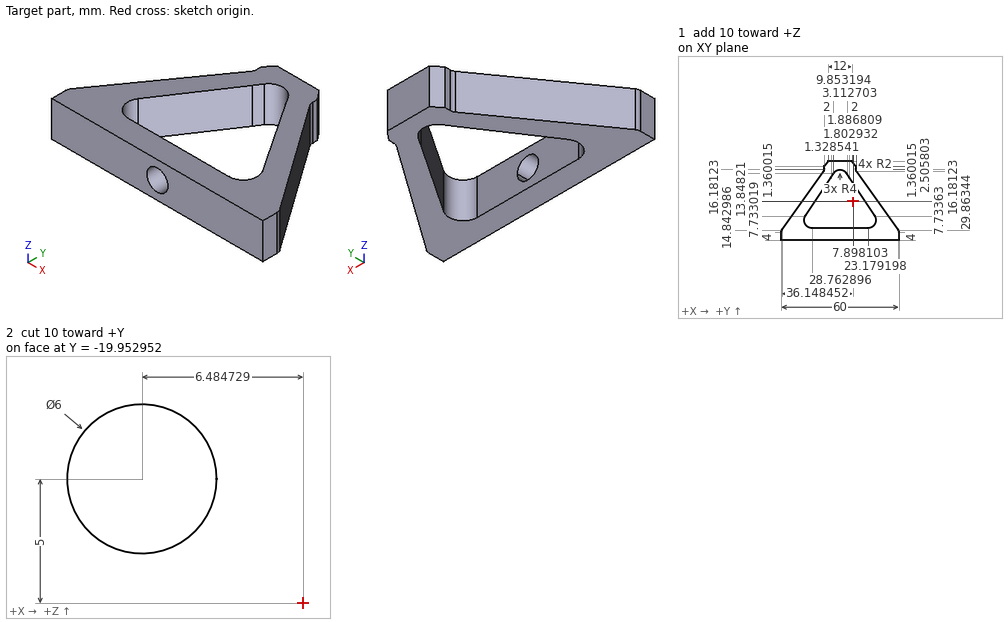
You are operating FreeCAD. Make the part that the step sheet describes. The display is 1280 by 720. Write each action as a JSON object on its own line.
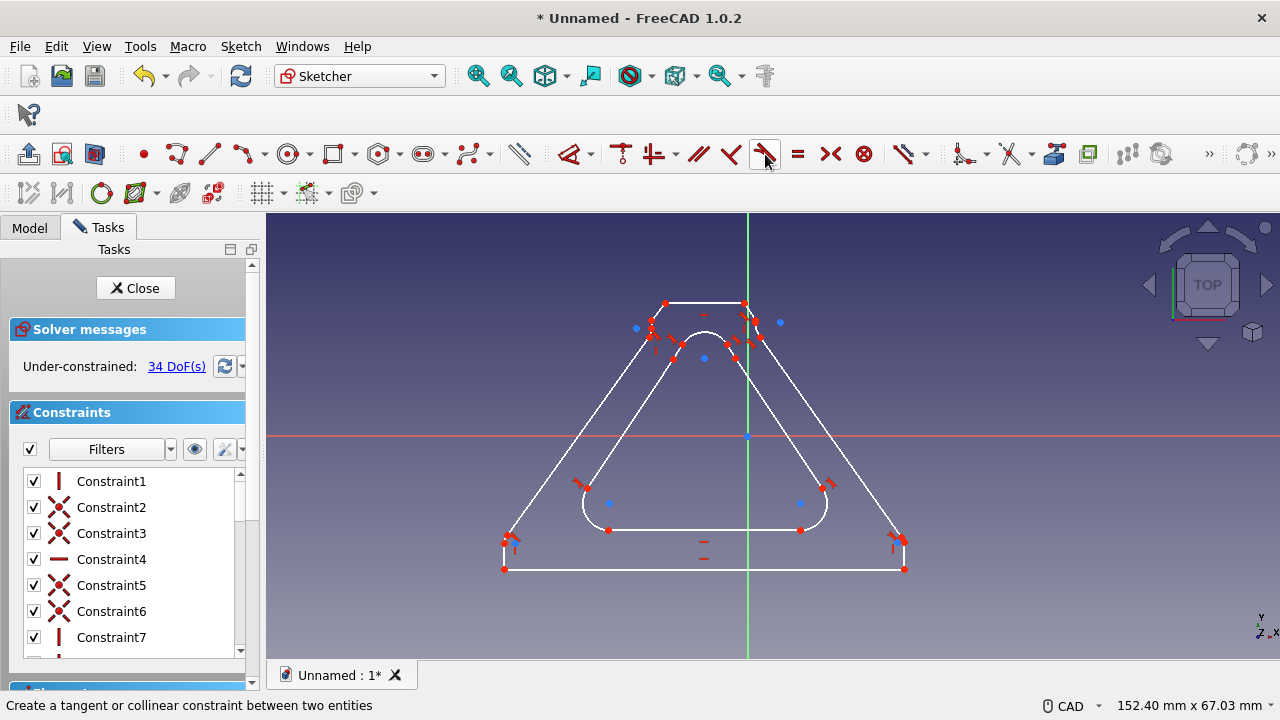
{"action": "left_click", "coordinate": [666, 530]}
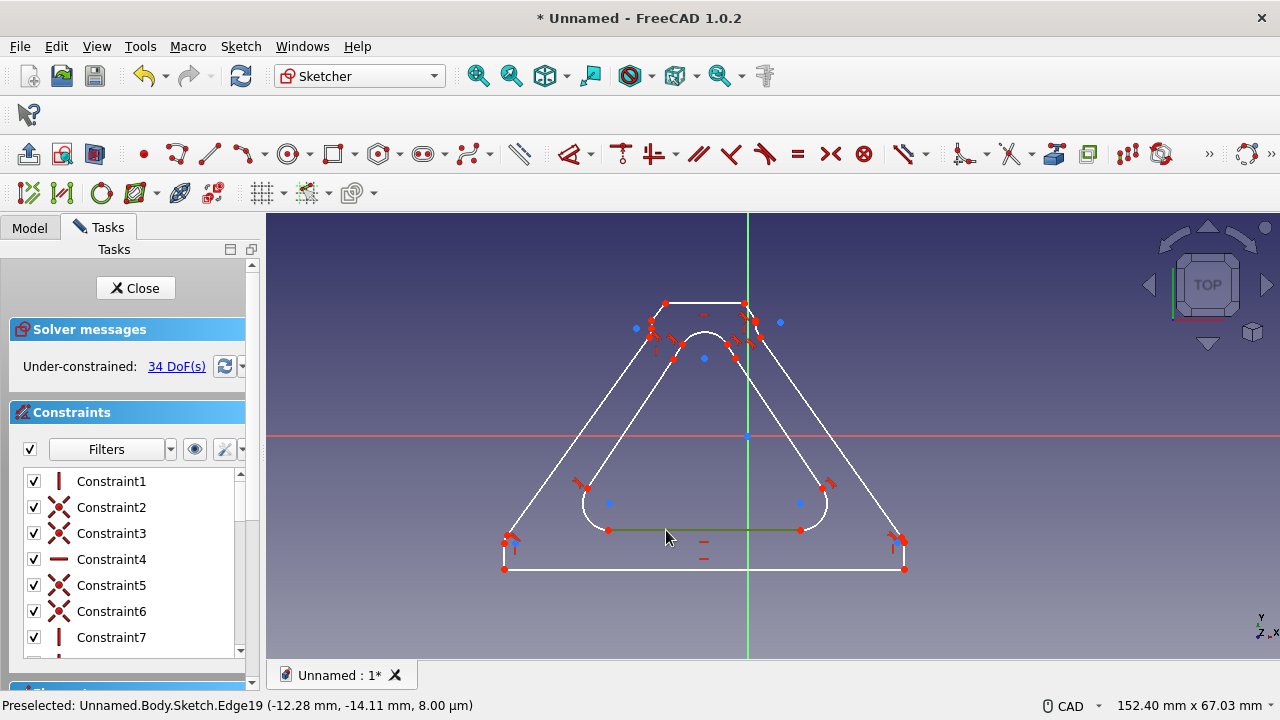
{"action": "left_click", "coordinate": [816, 525]}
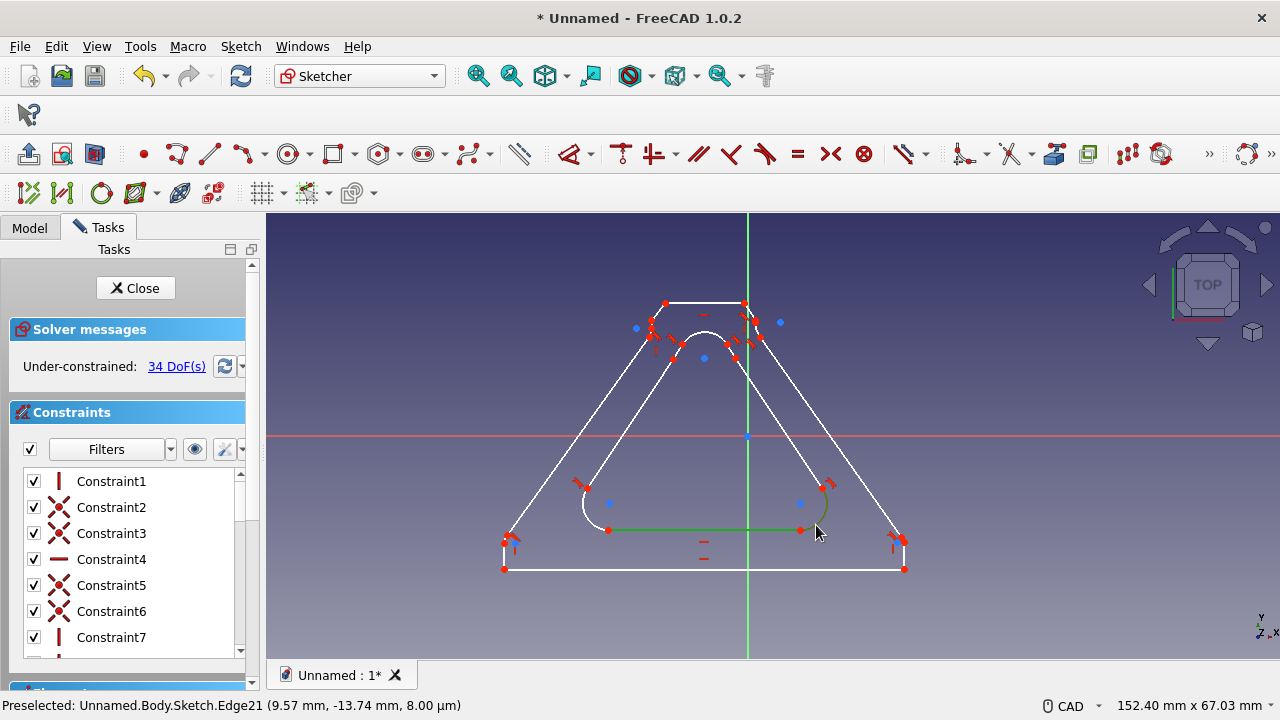
{"action": "left_click", "coordinate": [765, 154]}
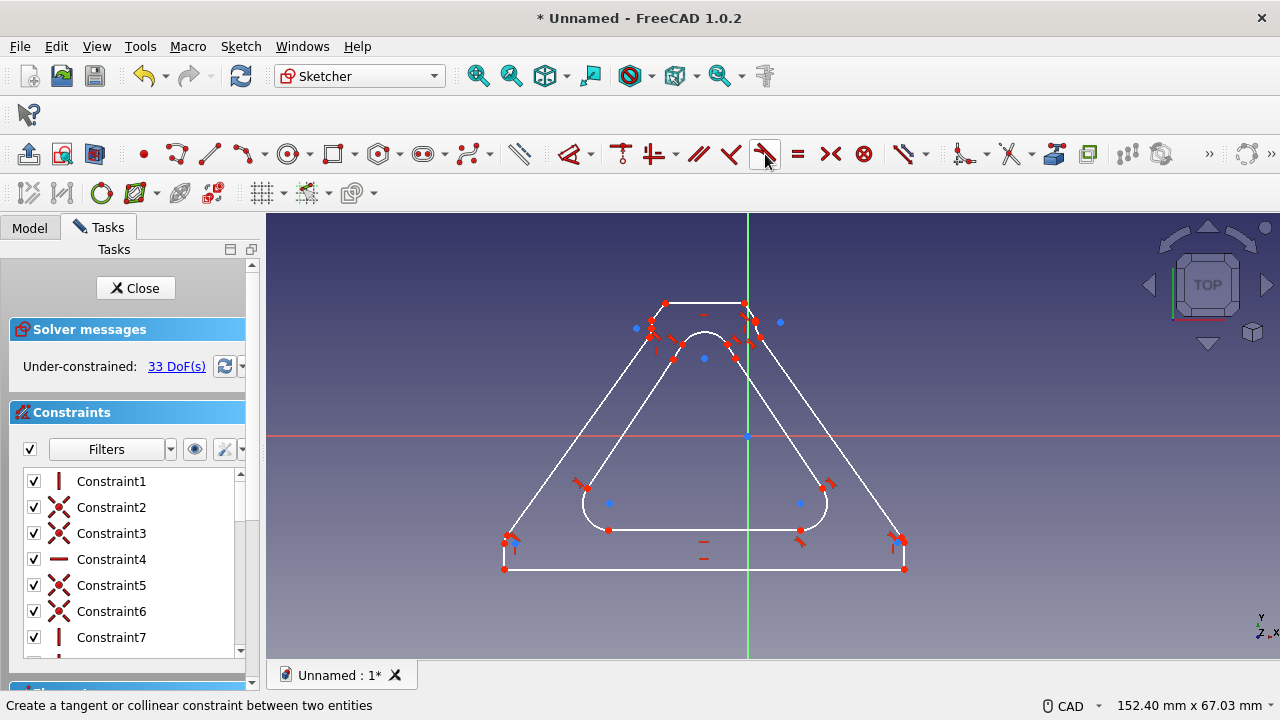
{"action": "left_click", "coordinate": [666, 530]}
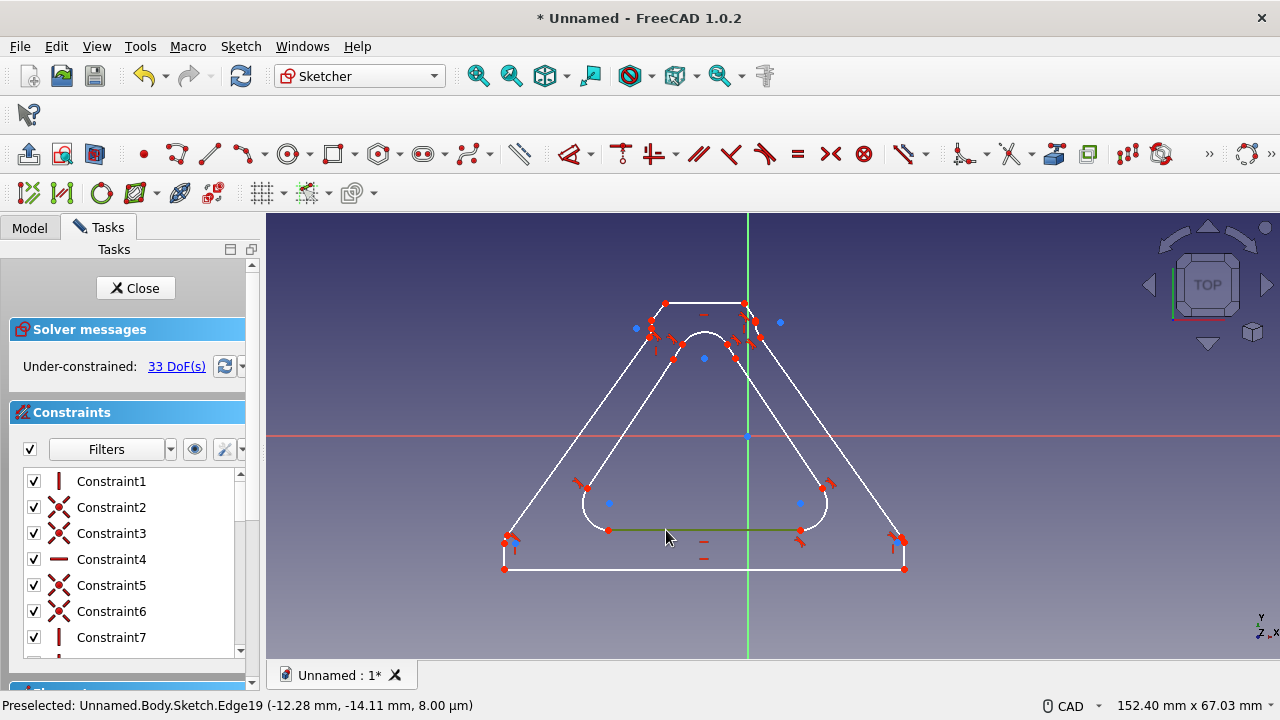
{"action": "left_click", "coordinate": [583, 505]}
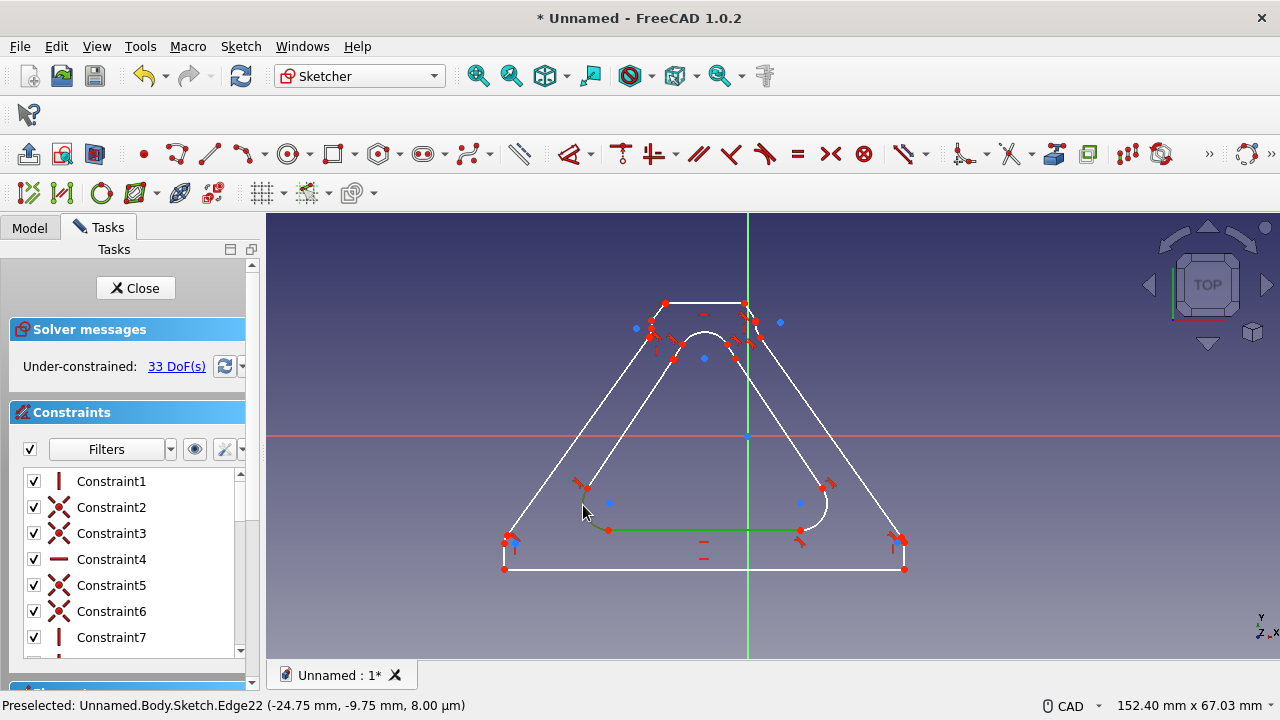
{"action": "left_click", "coordinate": [765, 154]}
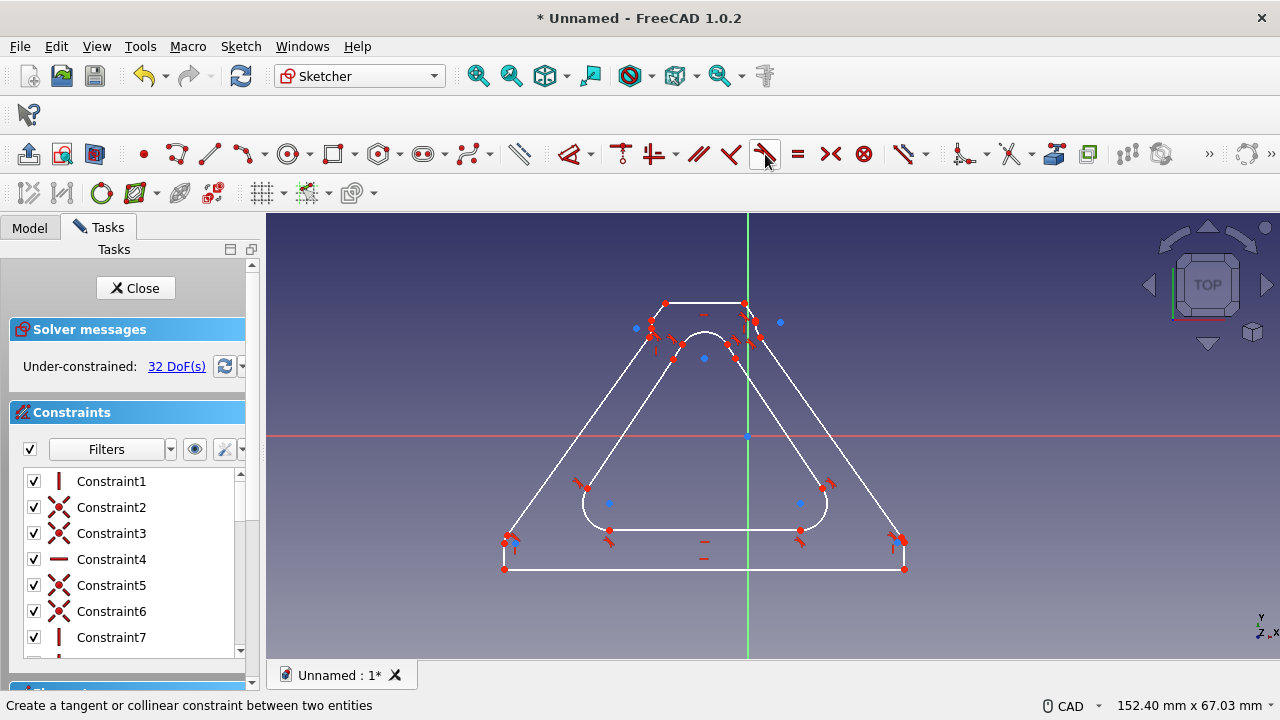
{"action": "scroll", "coordinate": [757, 330], "scroll_direction": "up", "scroll_amount": 3}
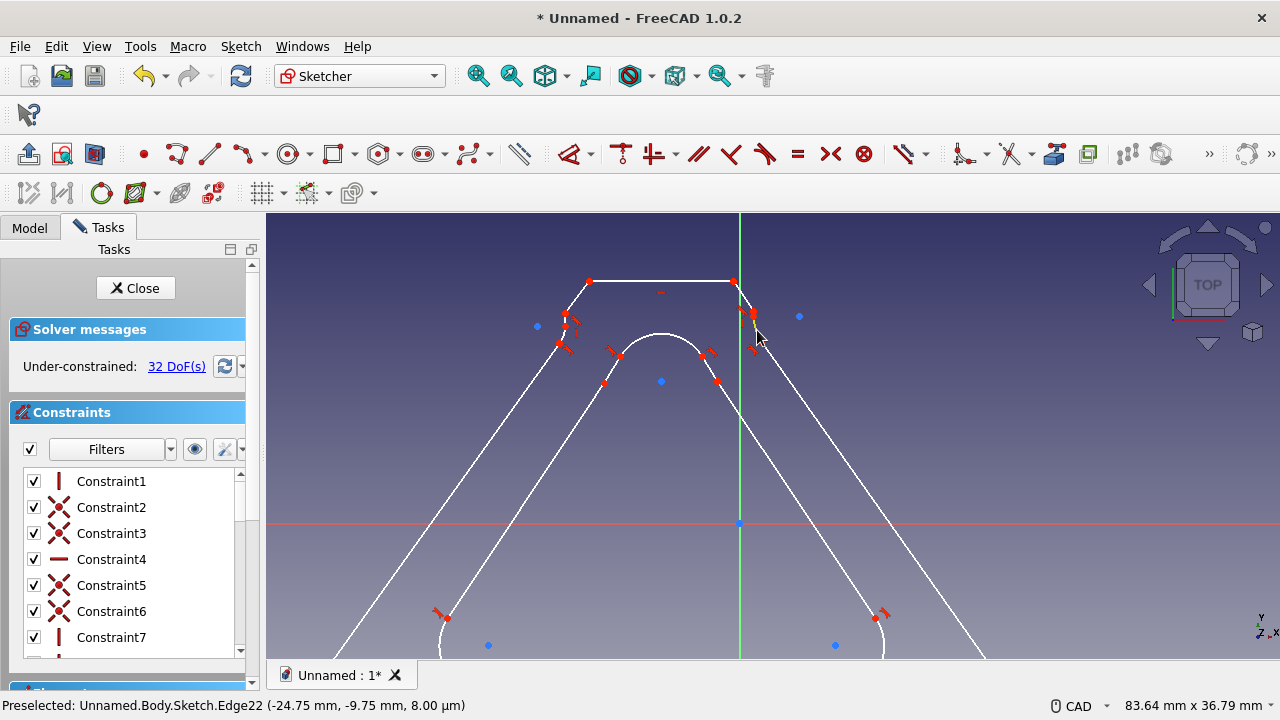
{"action": "left_click", "coordinate": [756, 330]}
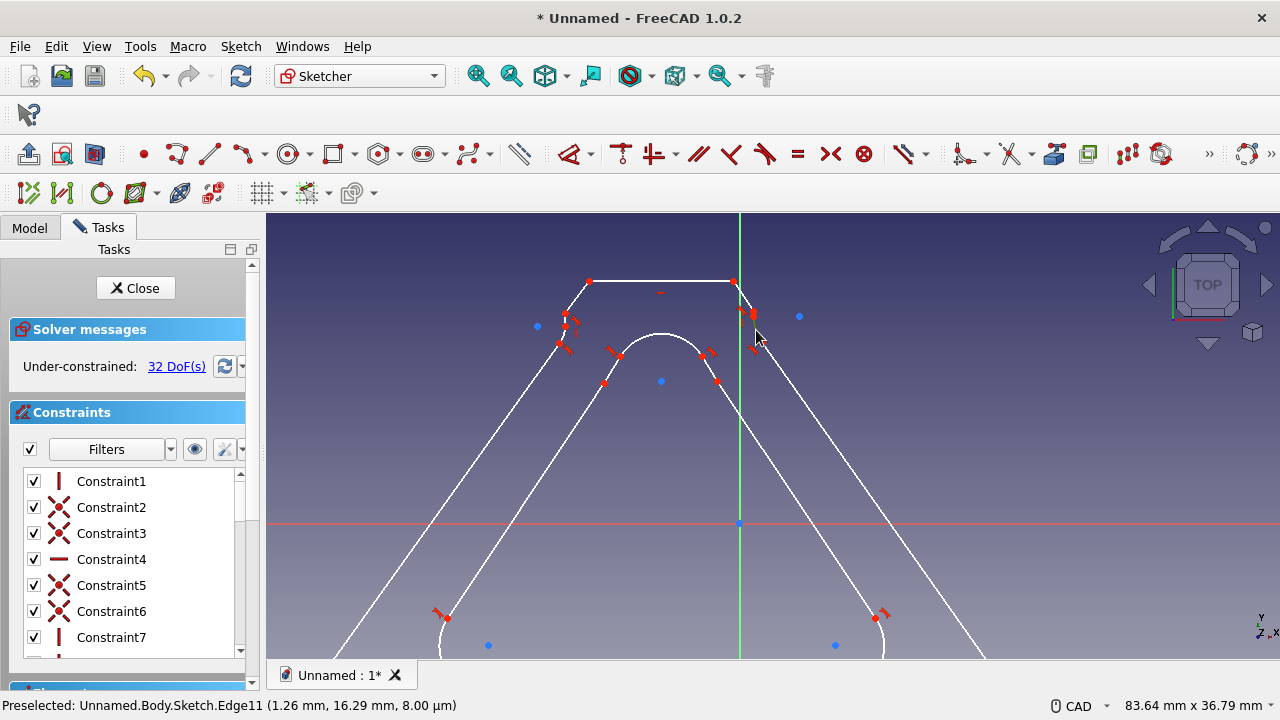
{"action": "scroll", "coordinate": [564, 335], "scroll_direction": "up", "scroll_amount": 3}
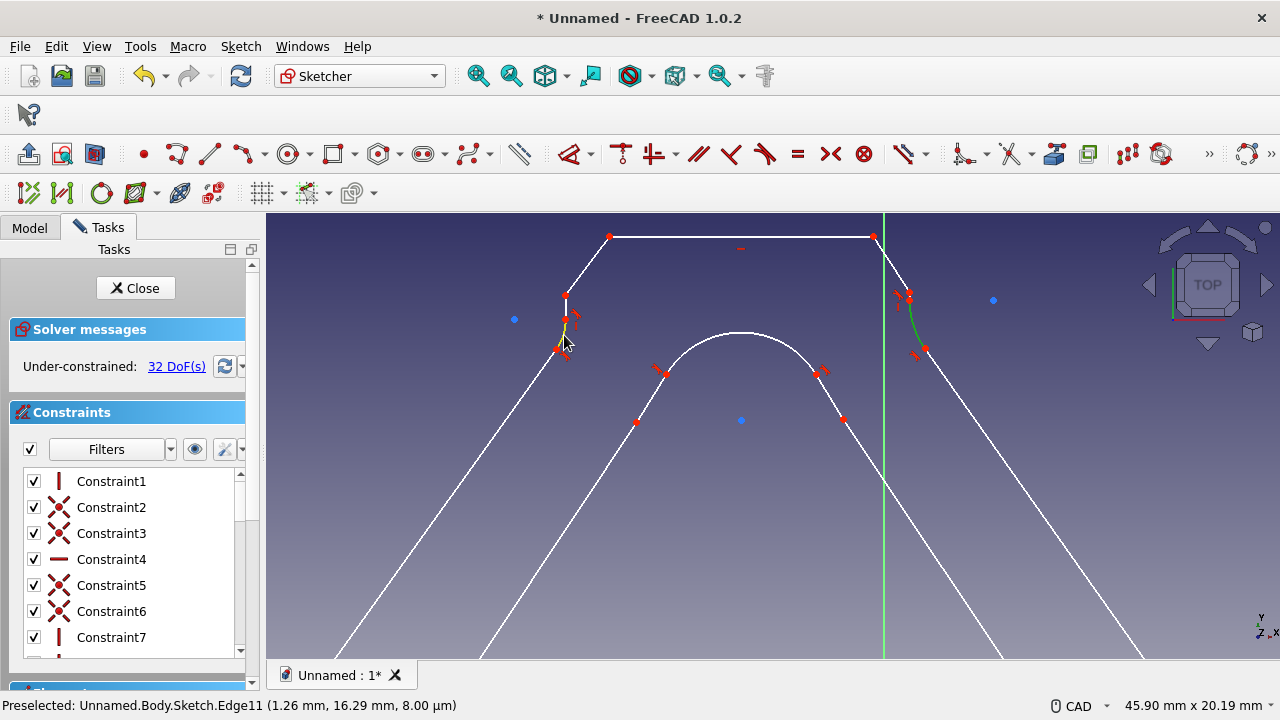
{"action": "left_click", "coordinate": [563, 335]}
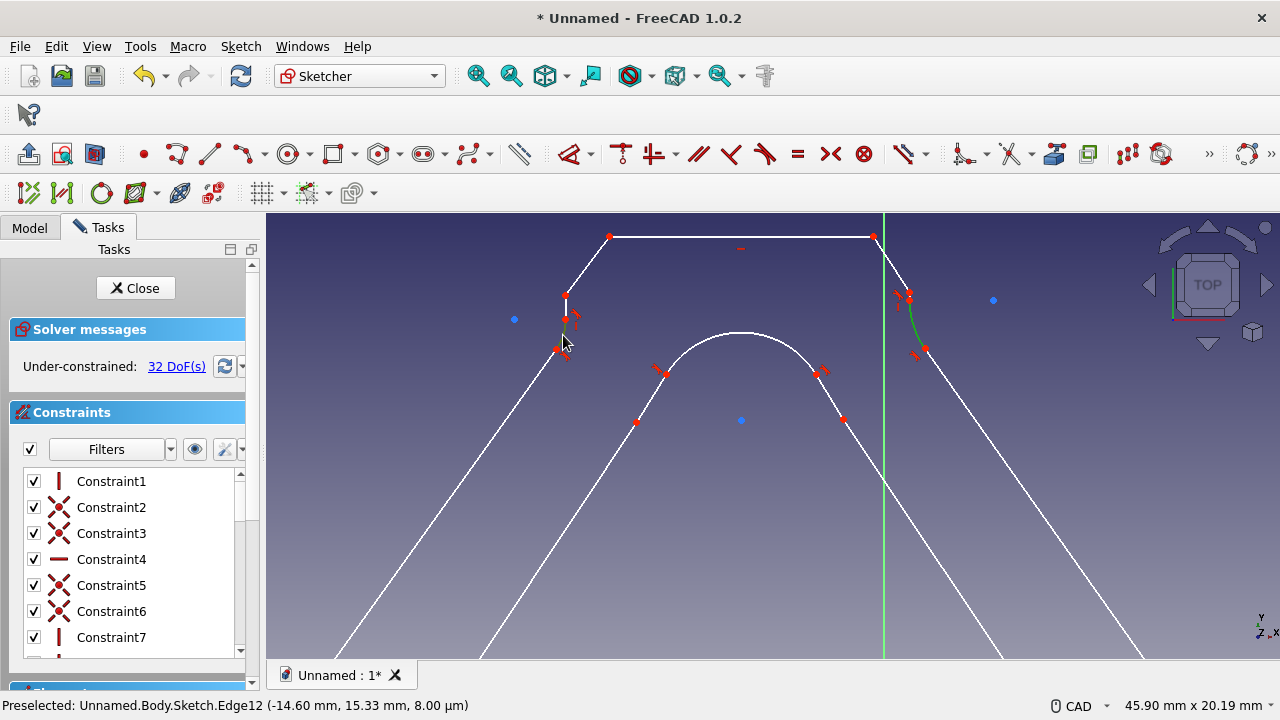
{"action": "scroll", "coordinate": [689, 332], "scroll_direction": "down", "scroll_amount": 6}